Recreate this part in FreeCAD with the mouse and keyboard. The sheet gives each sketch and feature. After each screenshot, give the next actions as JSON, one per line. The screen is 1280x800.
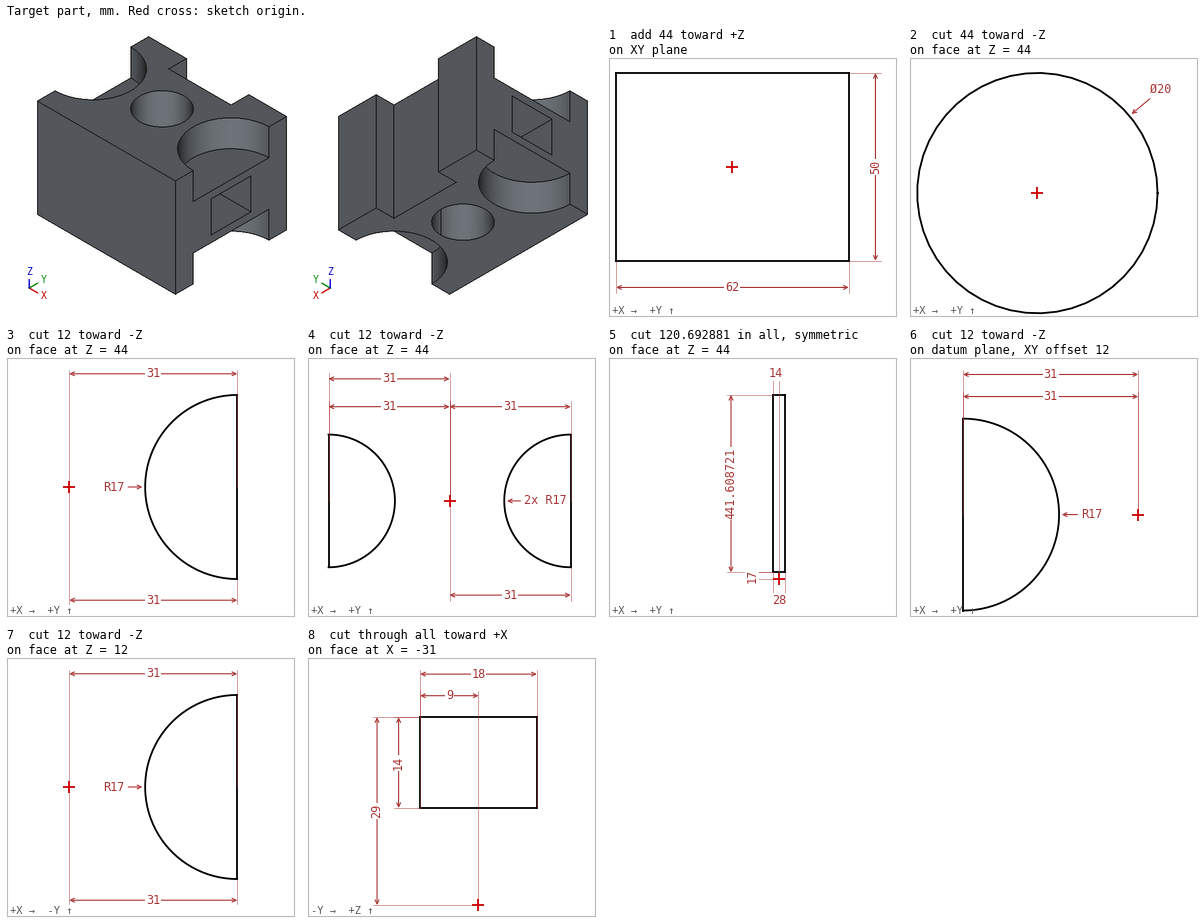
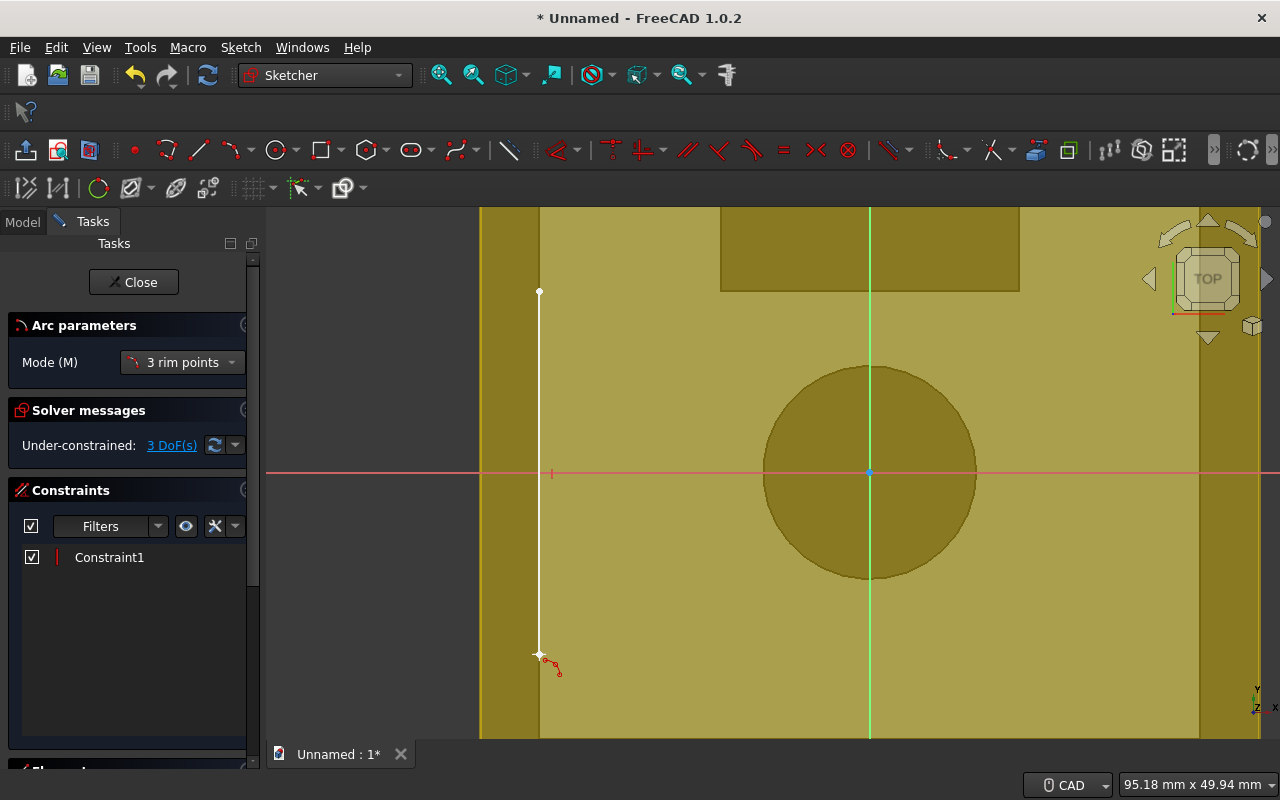
{"action": "left_click", "coordinate": [539, 655]}
{"action": "left_click", "coordinate": [539, 292]}
{"action": "left_click", "coordinate": [712, 529]}
{"action": "key", "text": "Escape"}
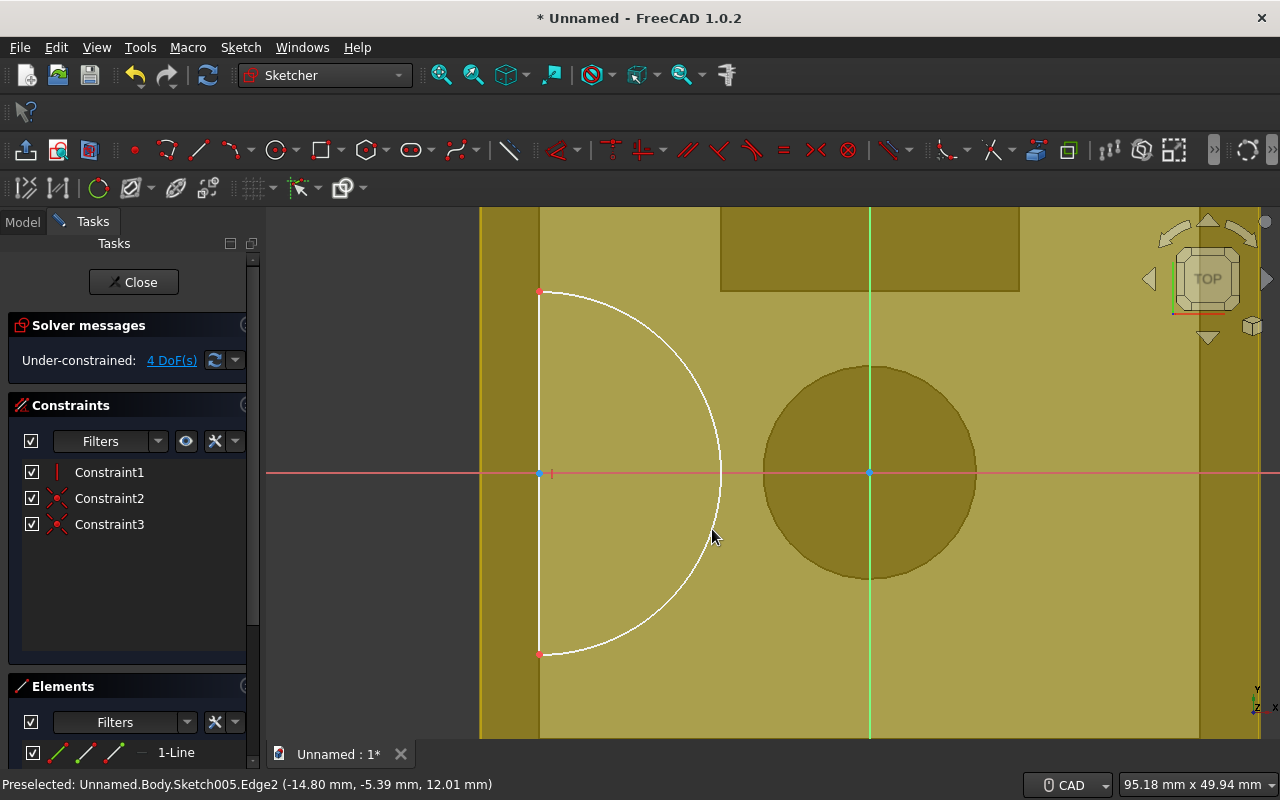
{"action": "left_click", "coordinate": [540, 473]}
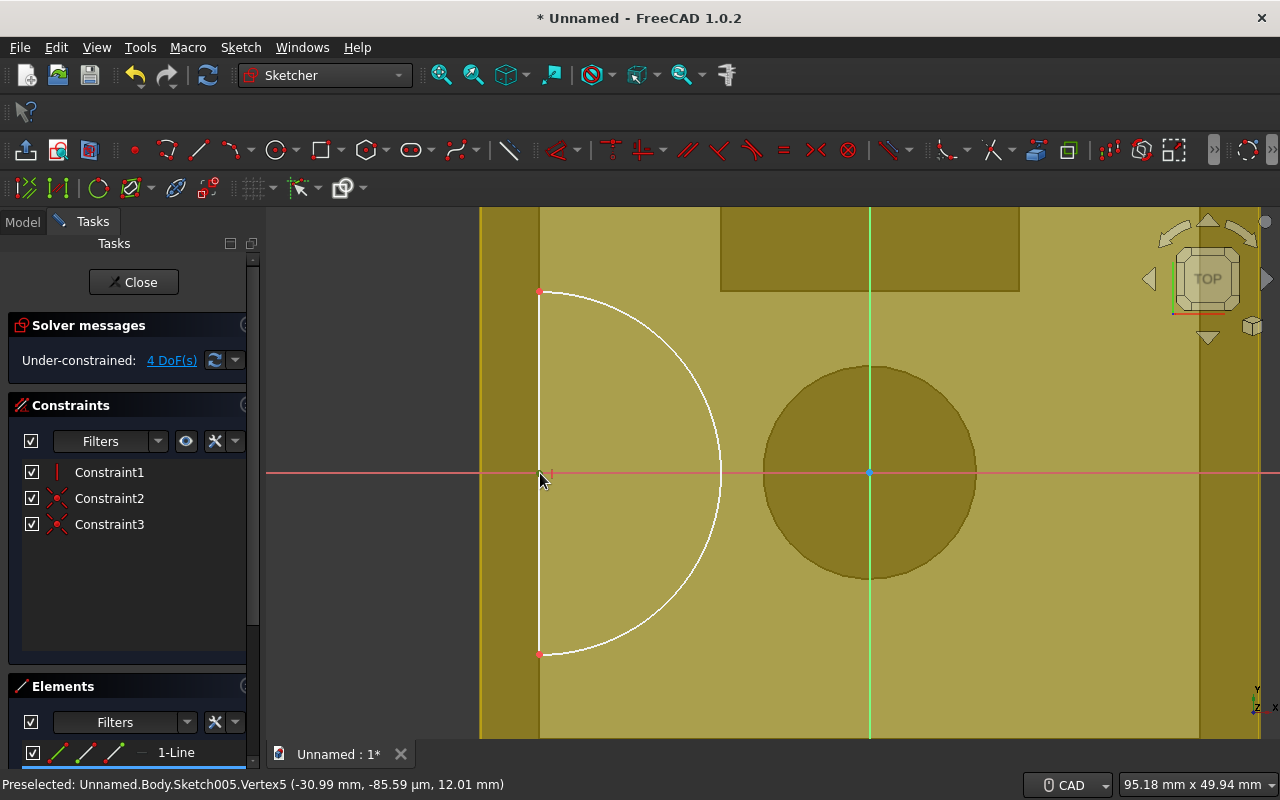
{"action": "left_click", "coordinate": [353, 473]}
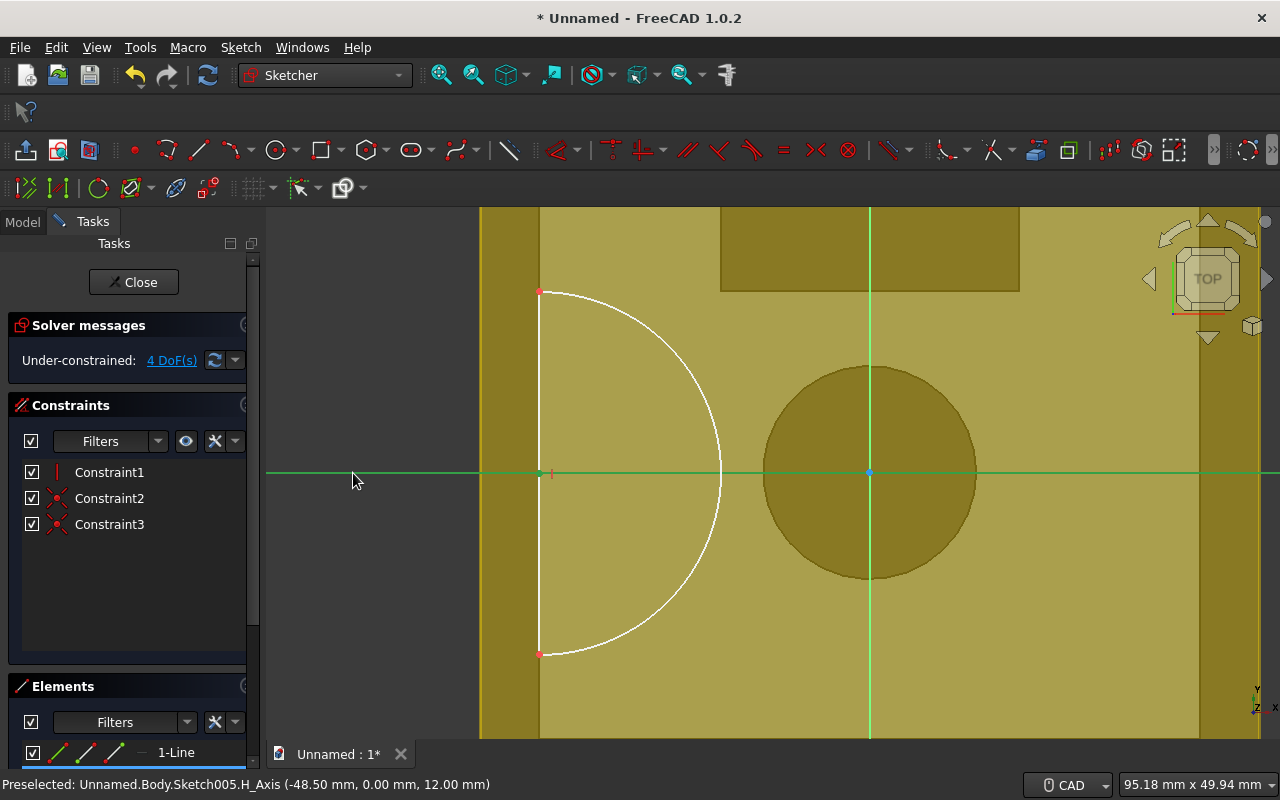
{"action": "left_click", "coordinate": [612, 150]}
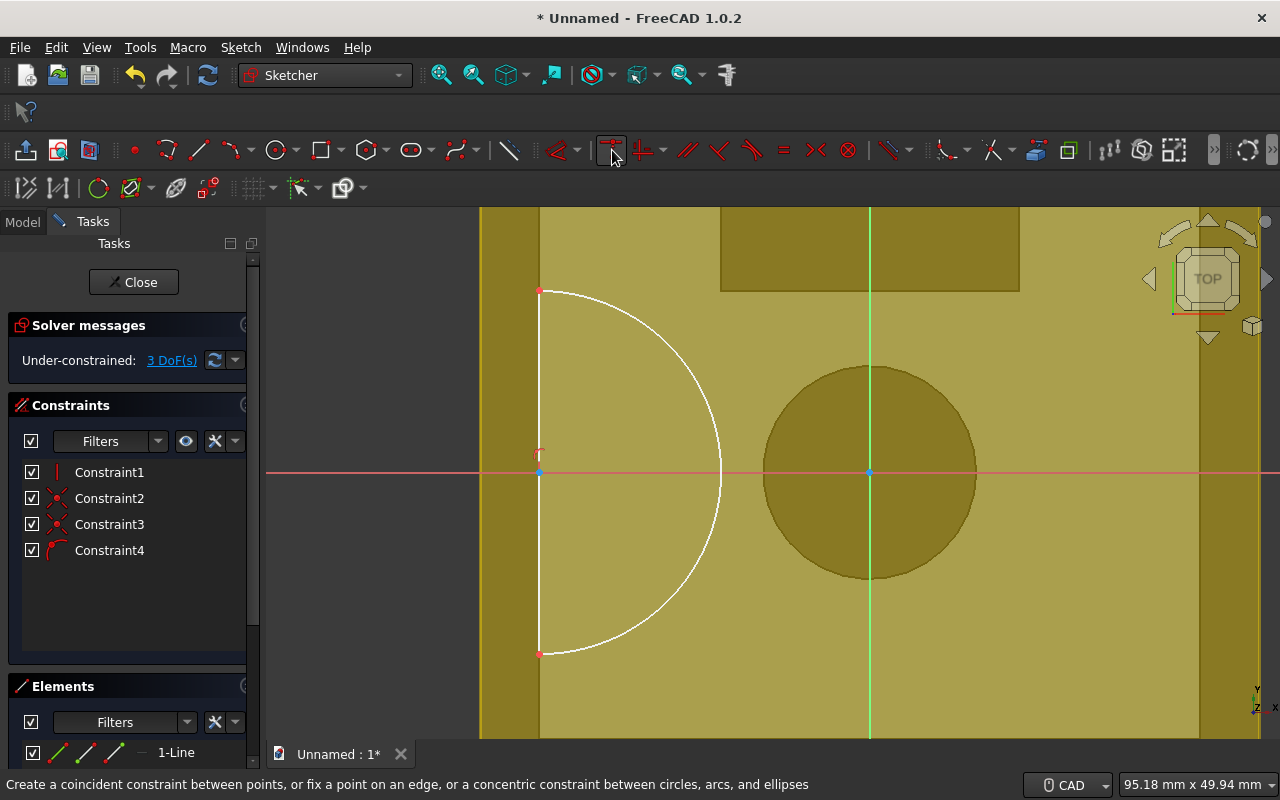
{"action": "key", "text": "d"}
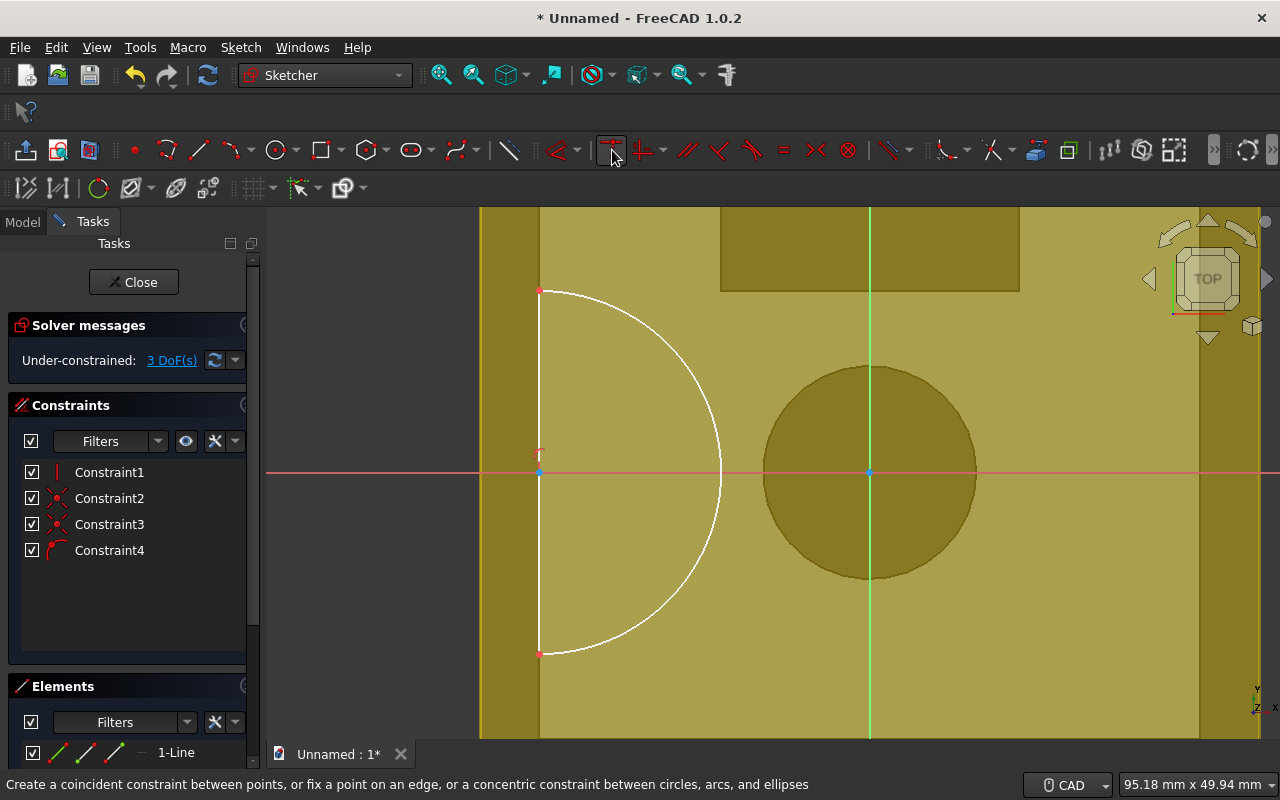
{"action": "left_click", "coordinate": [686, 580]}
{"action": "left_click", "coordinate": [712, 599]}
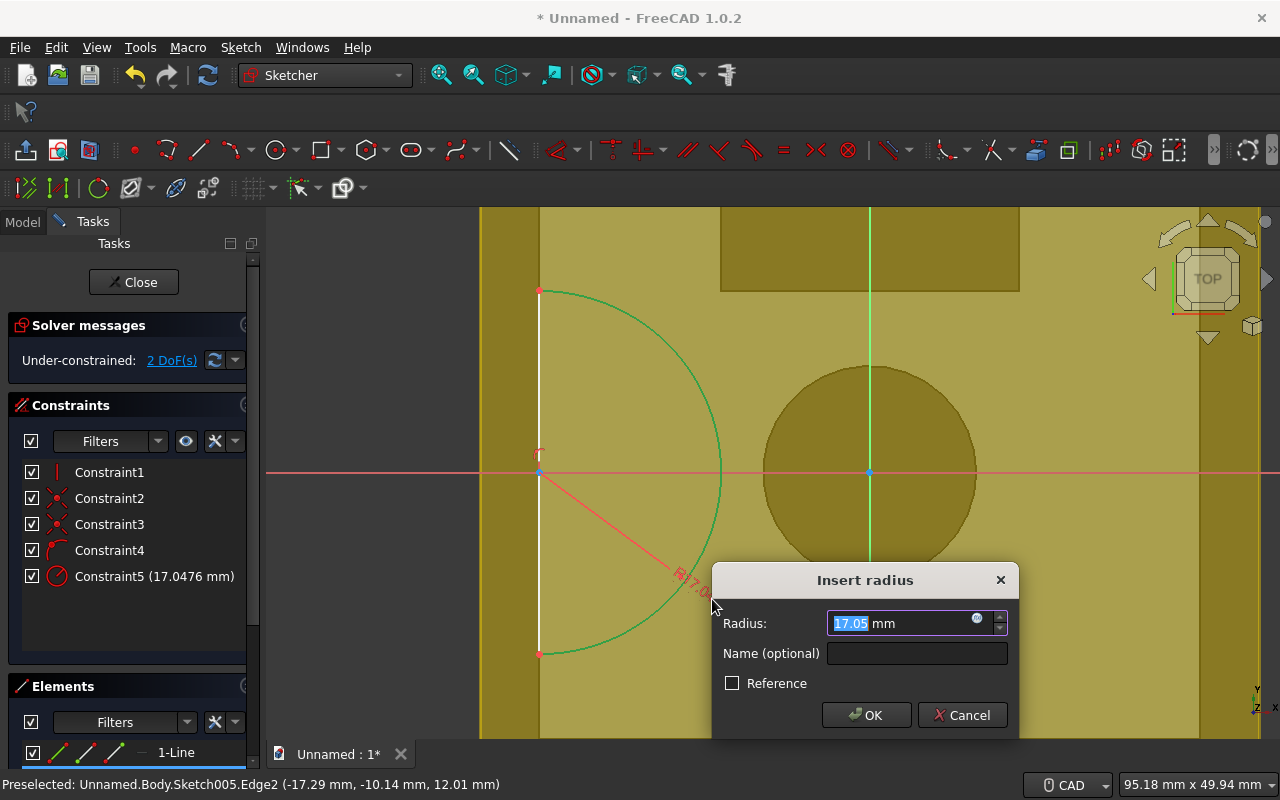
{"action": "type", "text": "17"}
{"action": "key", "text": "Return"}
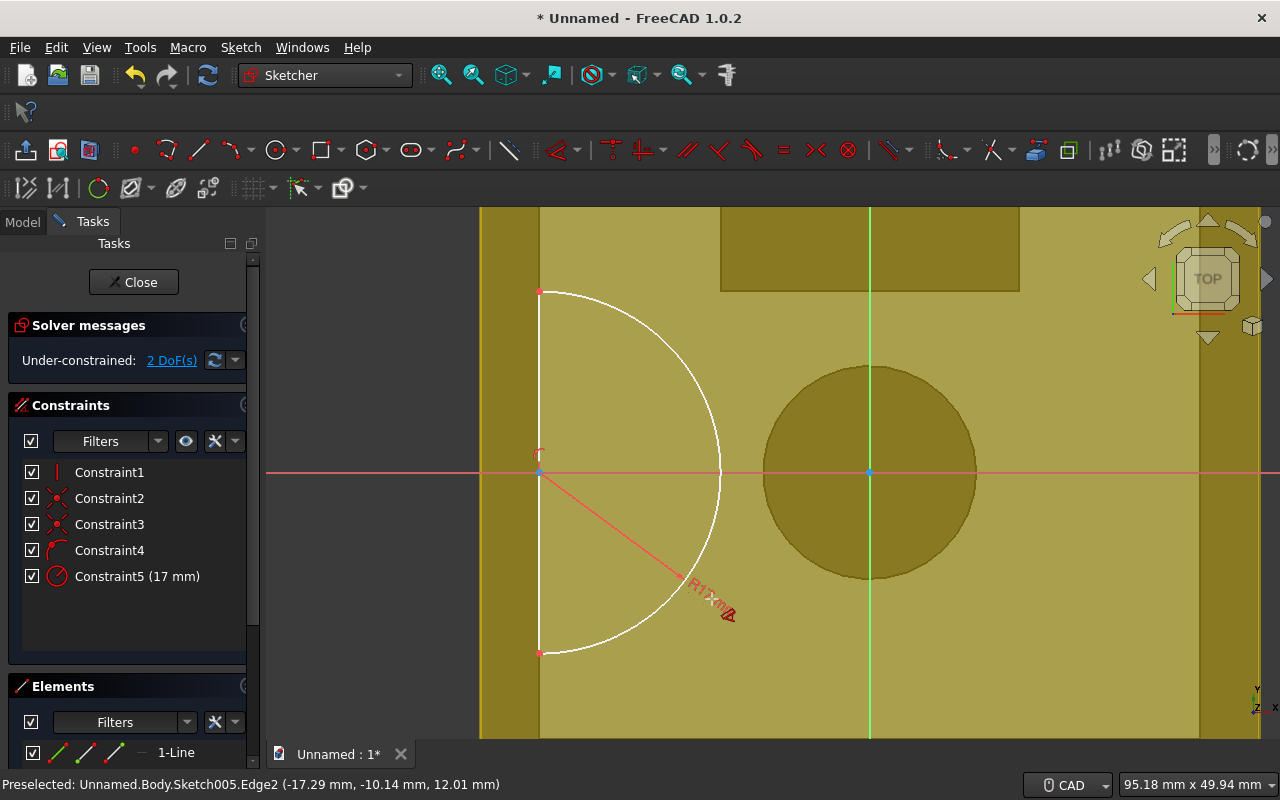
{"action": "left_click", "coordinate": [539, 291]}
{"action": "left_click", "coordinate": [704, 257]}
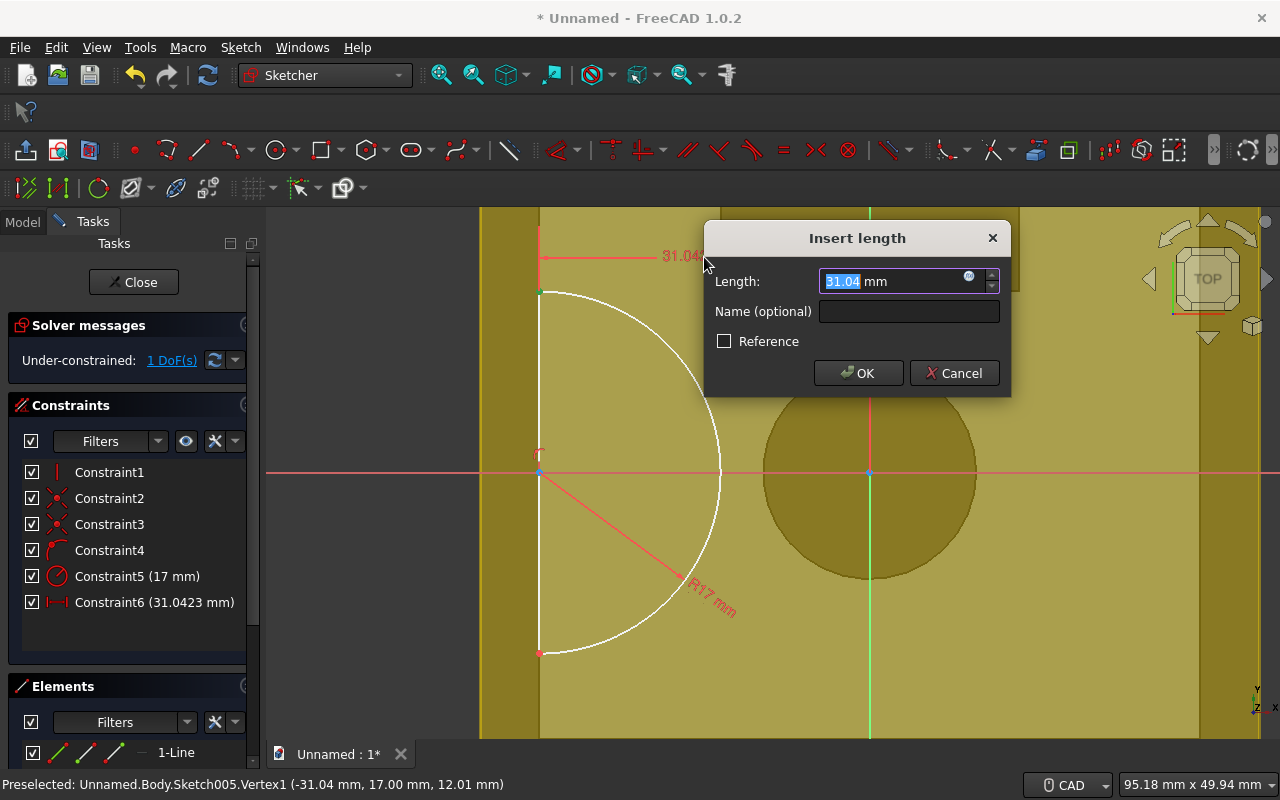
{"action": "type", "text": "31"}
{"action": "key", "text": "Return"}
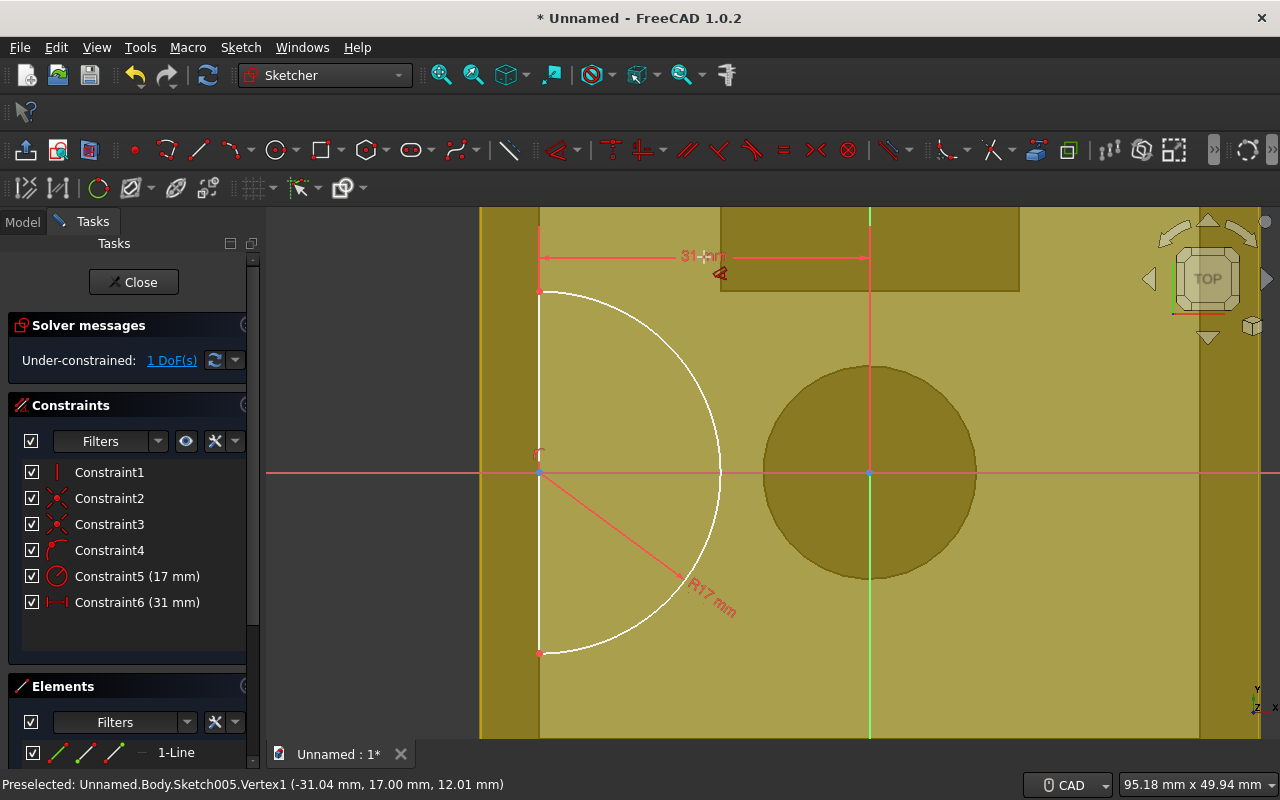
{"action": "left_click", "coordinate": [540, 473]}
{"action": "left_click", "coordinate": [629, 507]}